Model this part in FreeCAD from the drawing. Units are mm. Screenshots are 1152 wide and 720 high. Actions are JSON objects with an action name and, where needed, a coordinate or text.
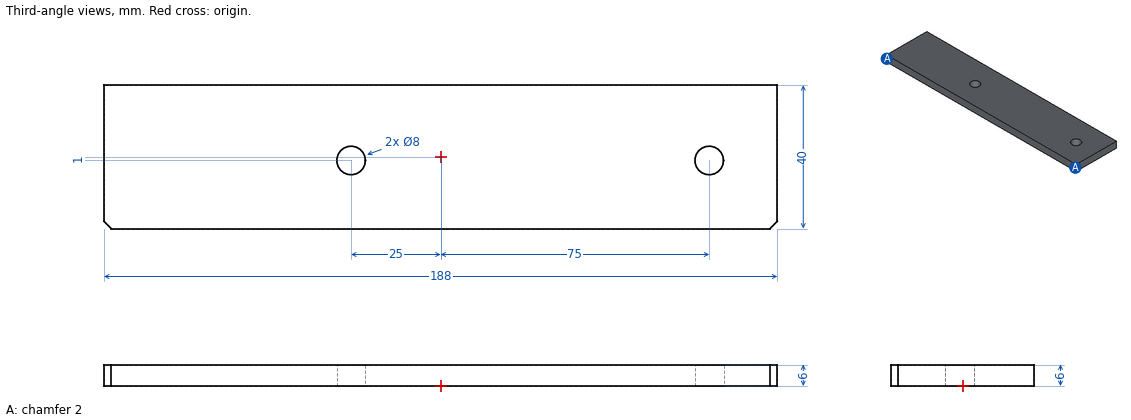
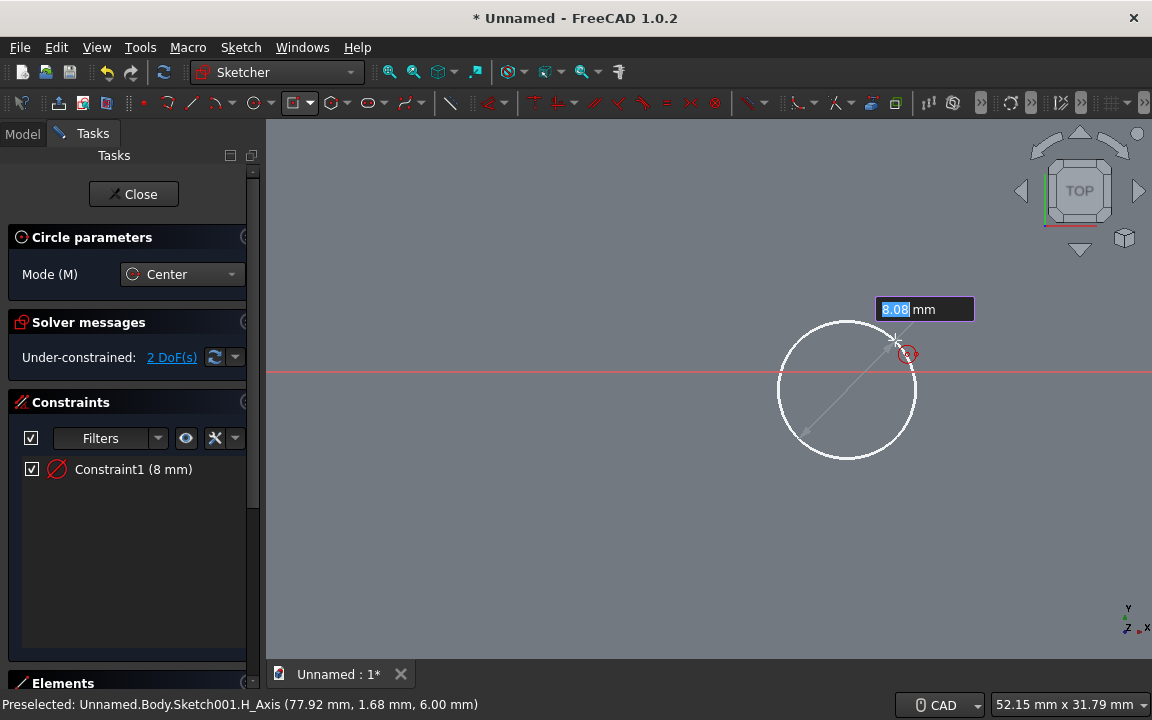
{"action": "type", "text": "8"}
{"action": "key", "text": "Return"}
{"action": "key", "text": "Escape"}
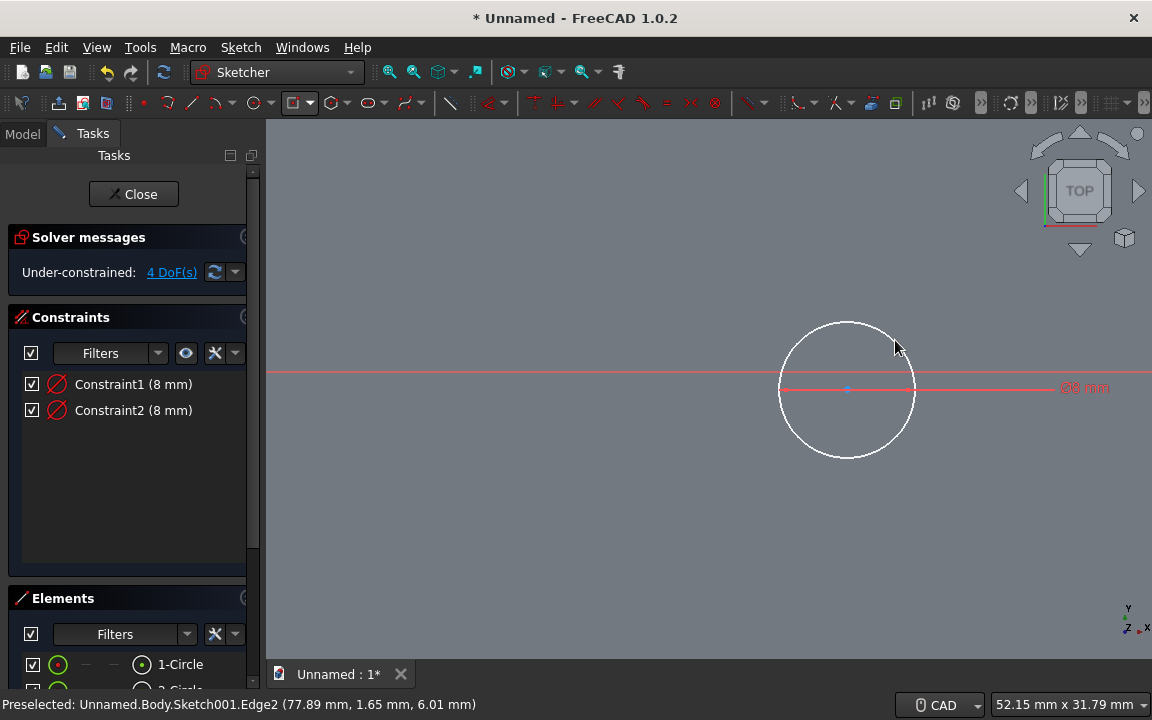
{"action": "scroll", "coordinate": [851, 389], "scroll_direction": "down", "scroll_amount": 7}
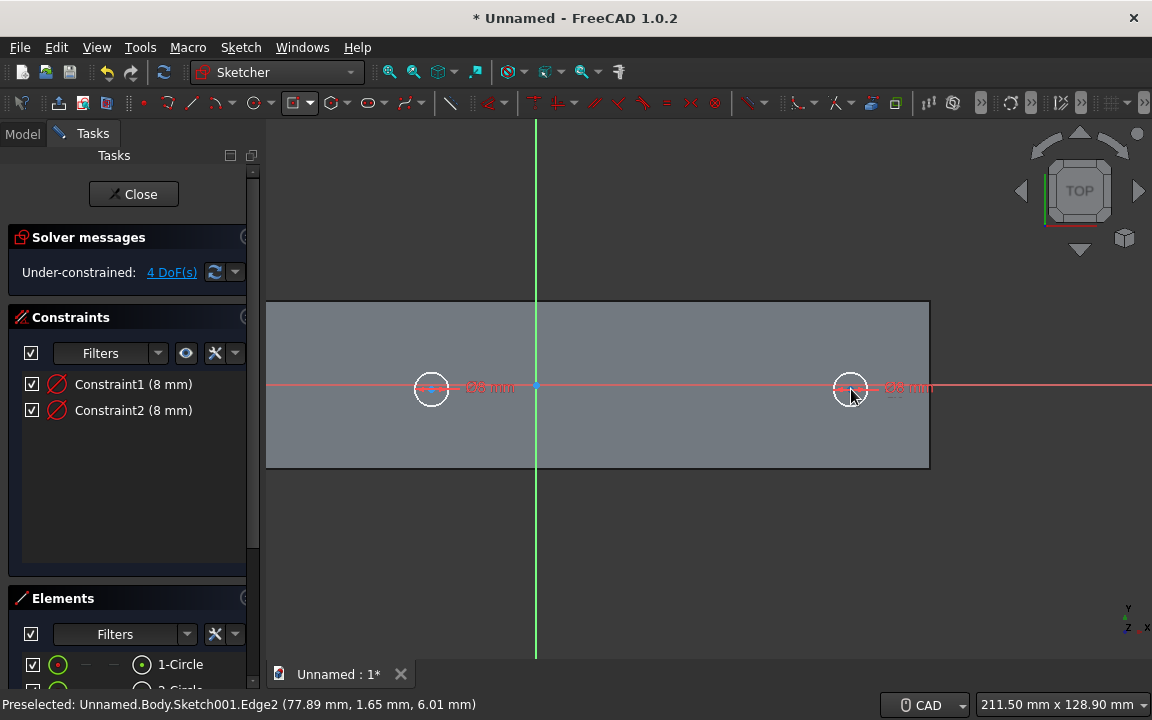
{"action": "left_click", "coordinate": [432, 389]}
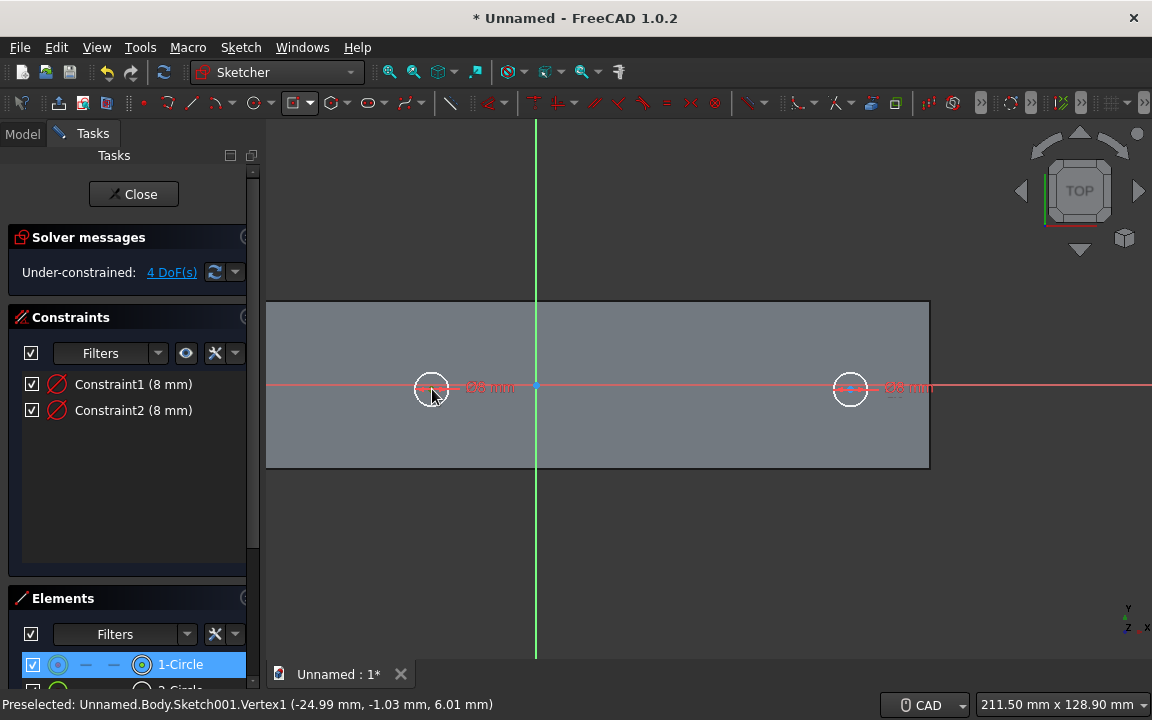
{"action": "left_click", "coordinate": [851, 390]}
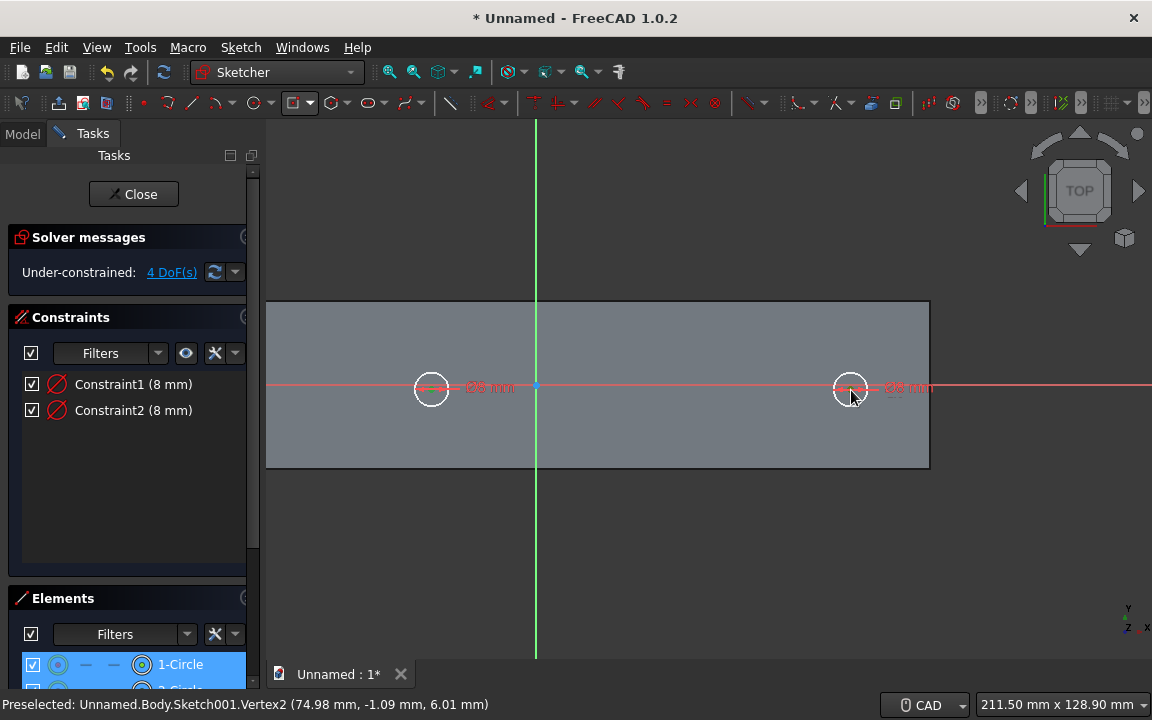
{"action": "key", "text": "h"}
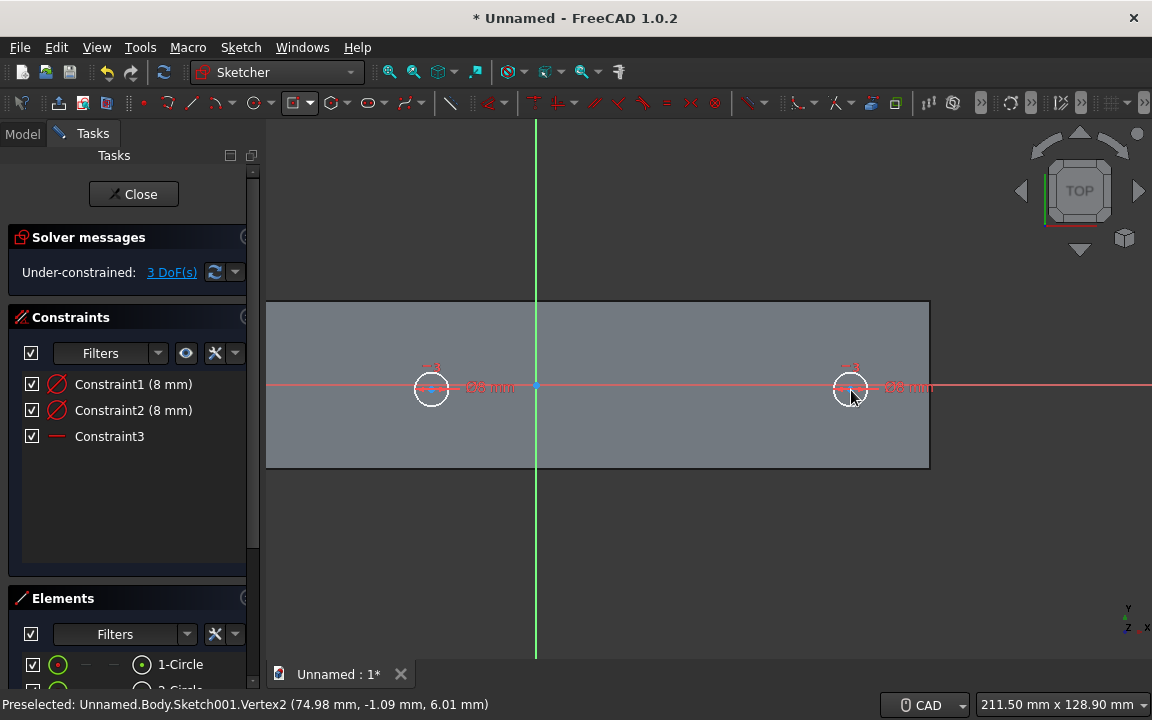
{"action": "scroll", "coordinate": [432, 389], "scroll_direction": "up", "scroll_amount": 12}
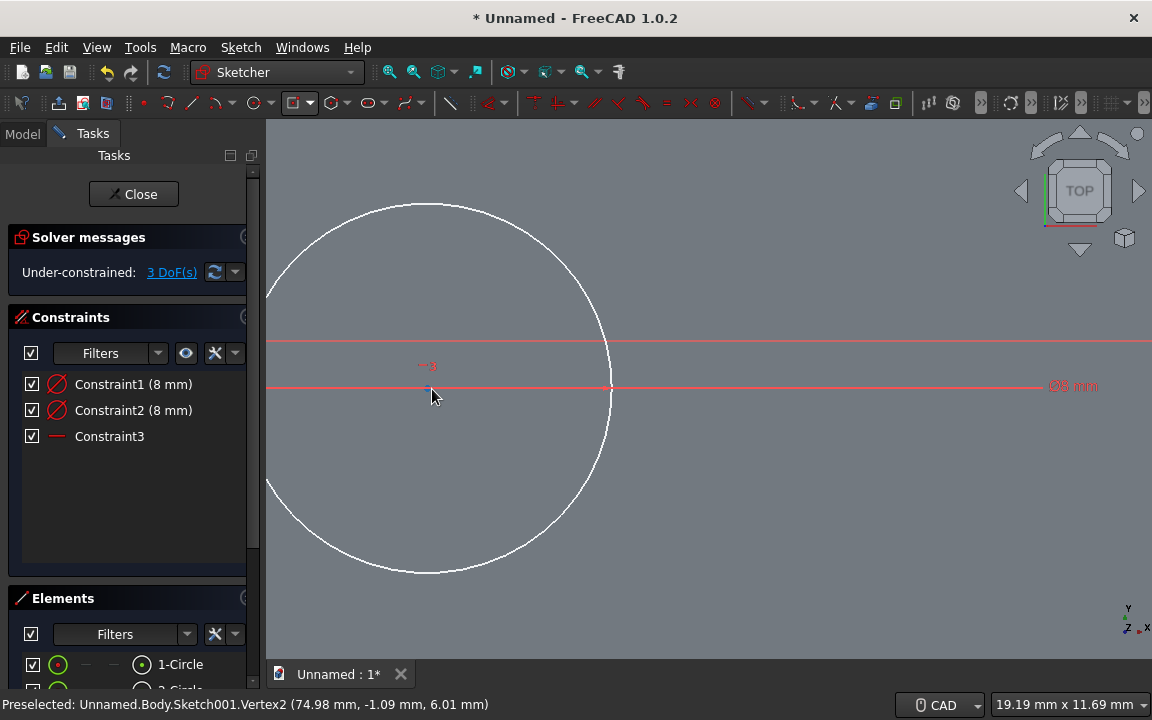
{"action": "left_click", "coordinate": [427, 388]}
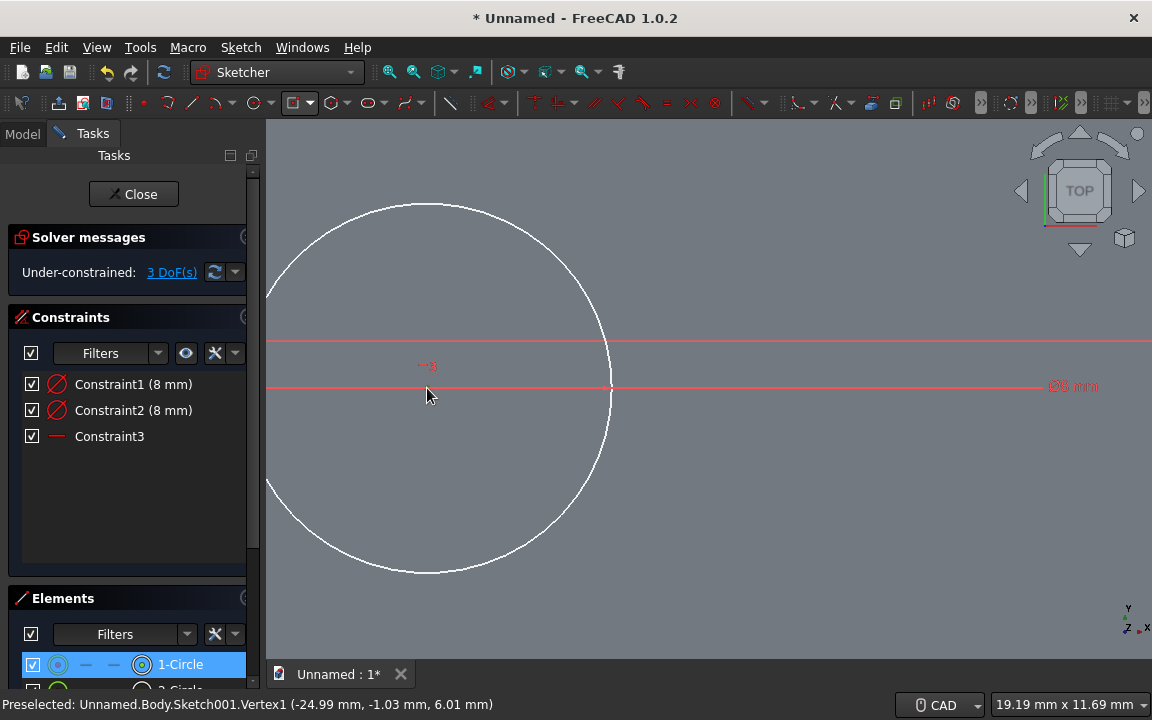
{"action": "left_click", "coordinate": [506, 104]}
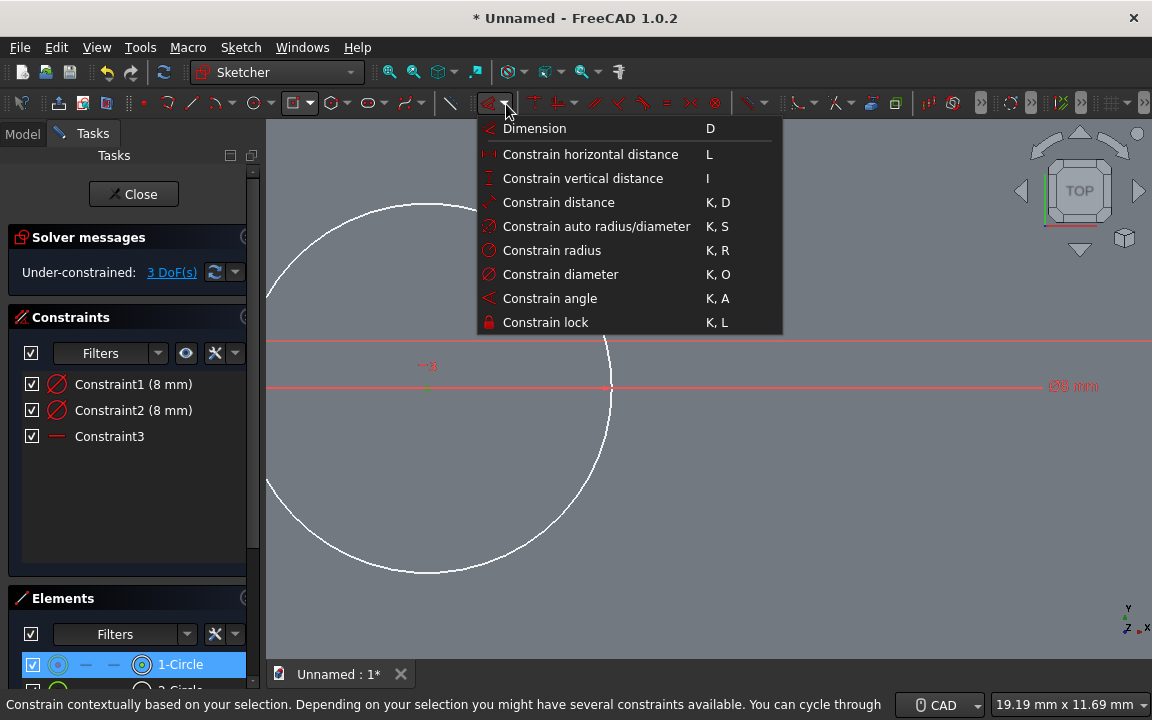
{"action": "left_click", "coordinate": [630, 178]}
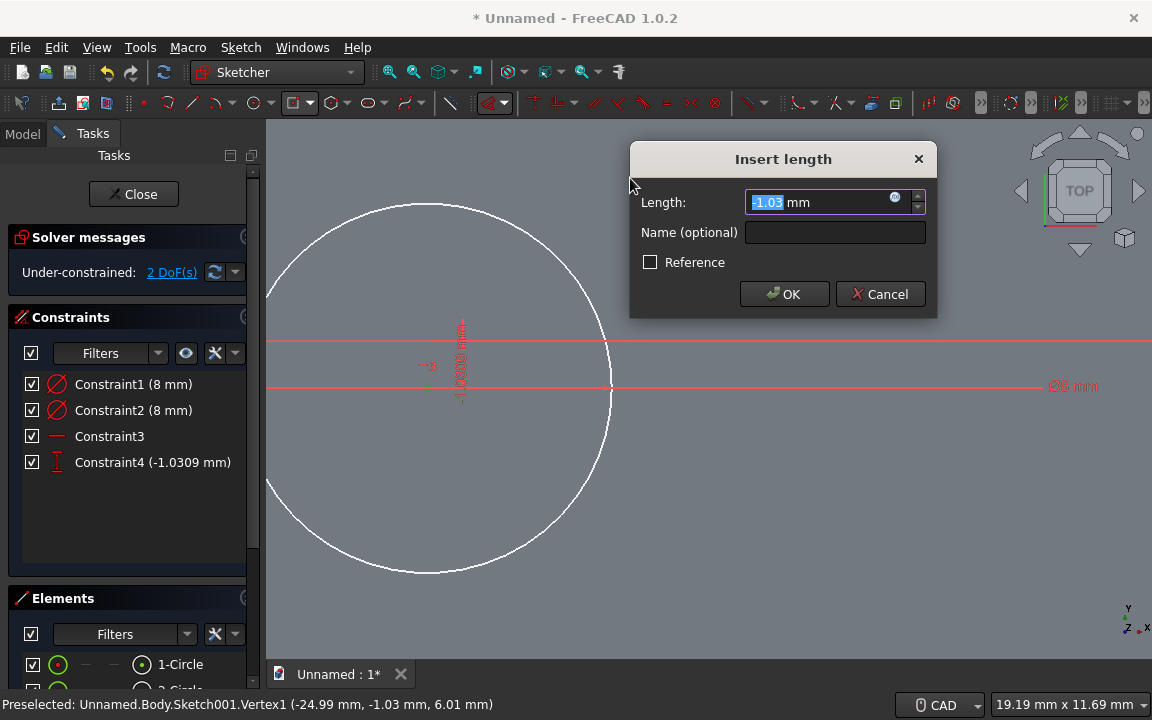
{"action": "type", "text": "-1"}
{"action": "key", "text": "Return"}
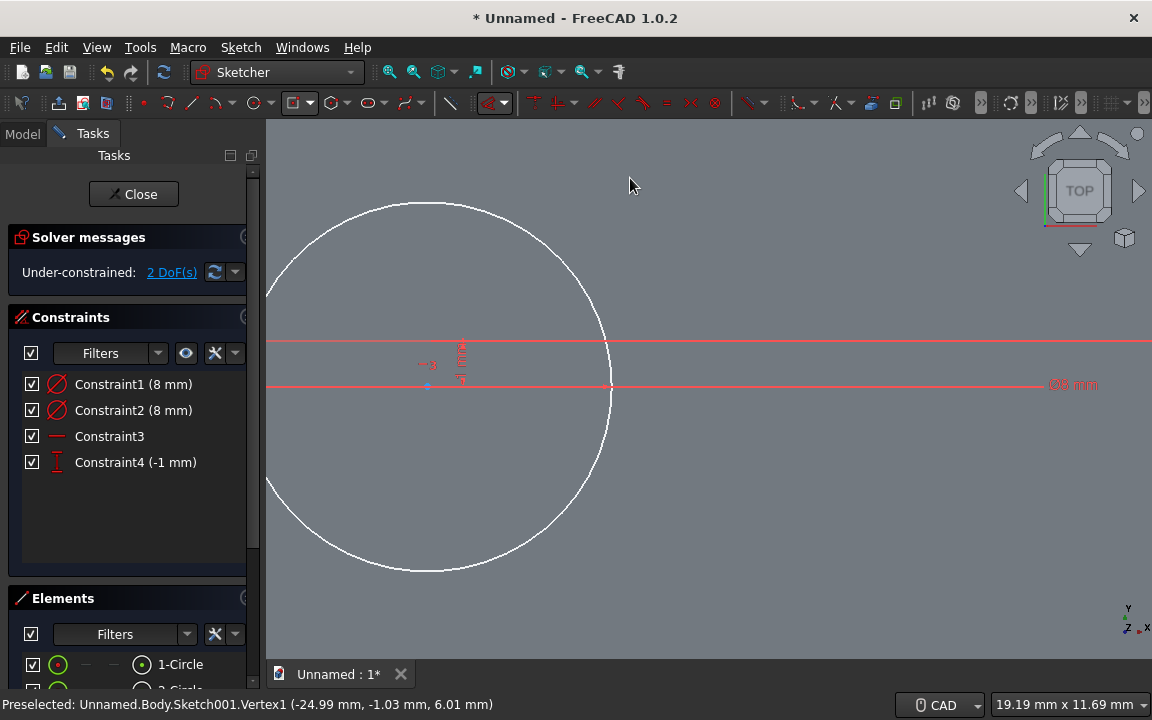
{"action": "scroll", "coordinate": [431, 389], "scroll_direction": "down", "scroll_amount": 12}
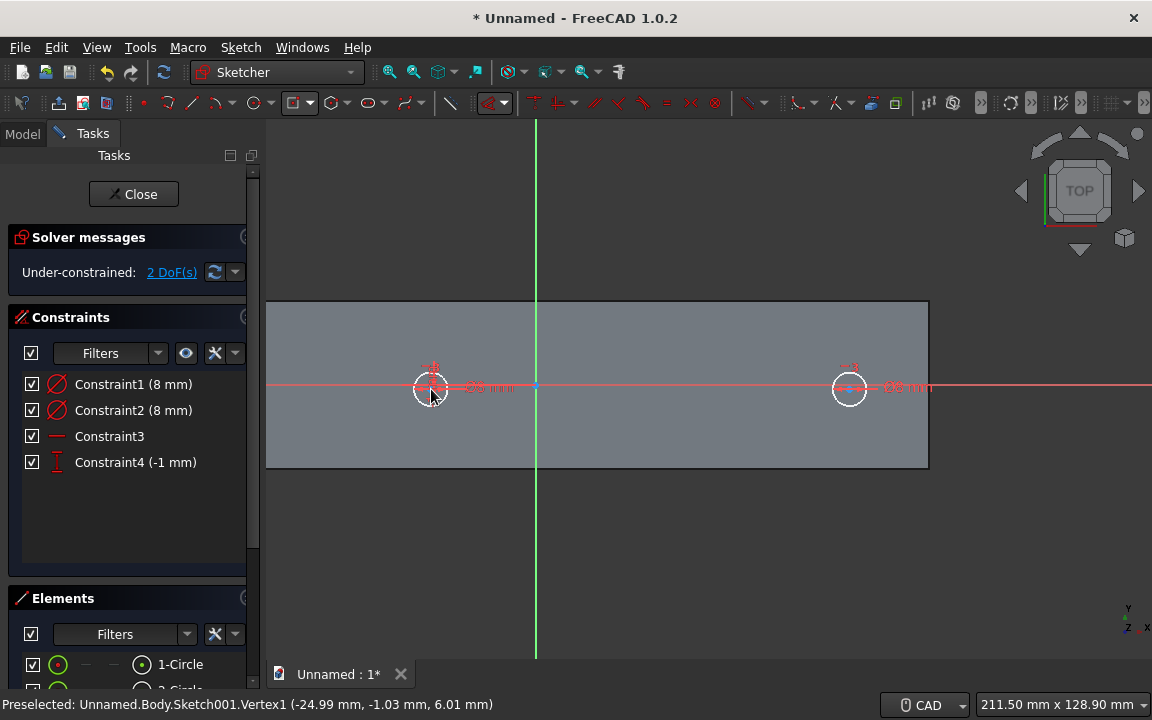
{"action": "left_click", "coordinate": [431, 389]}